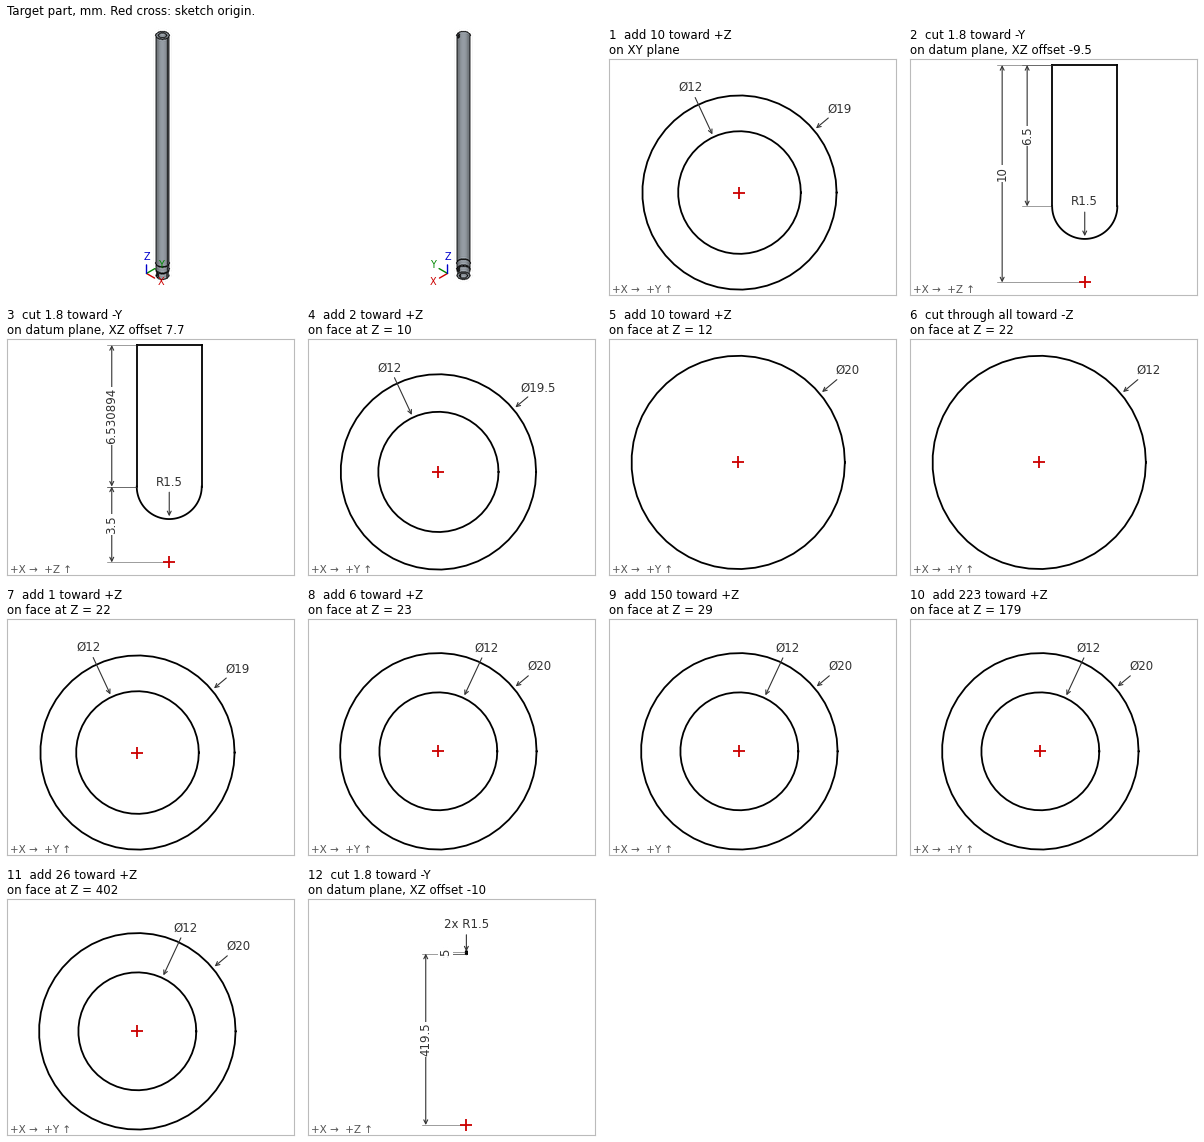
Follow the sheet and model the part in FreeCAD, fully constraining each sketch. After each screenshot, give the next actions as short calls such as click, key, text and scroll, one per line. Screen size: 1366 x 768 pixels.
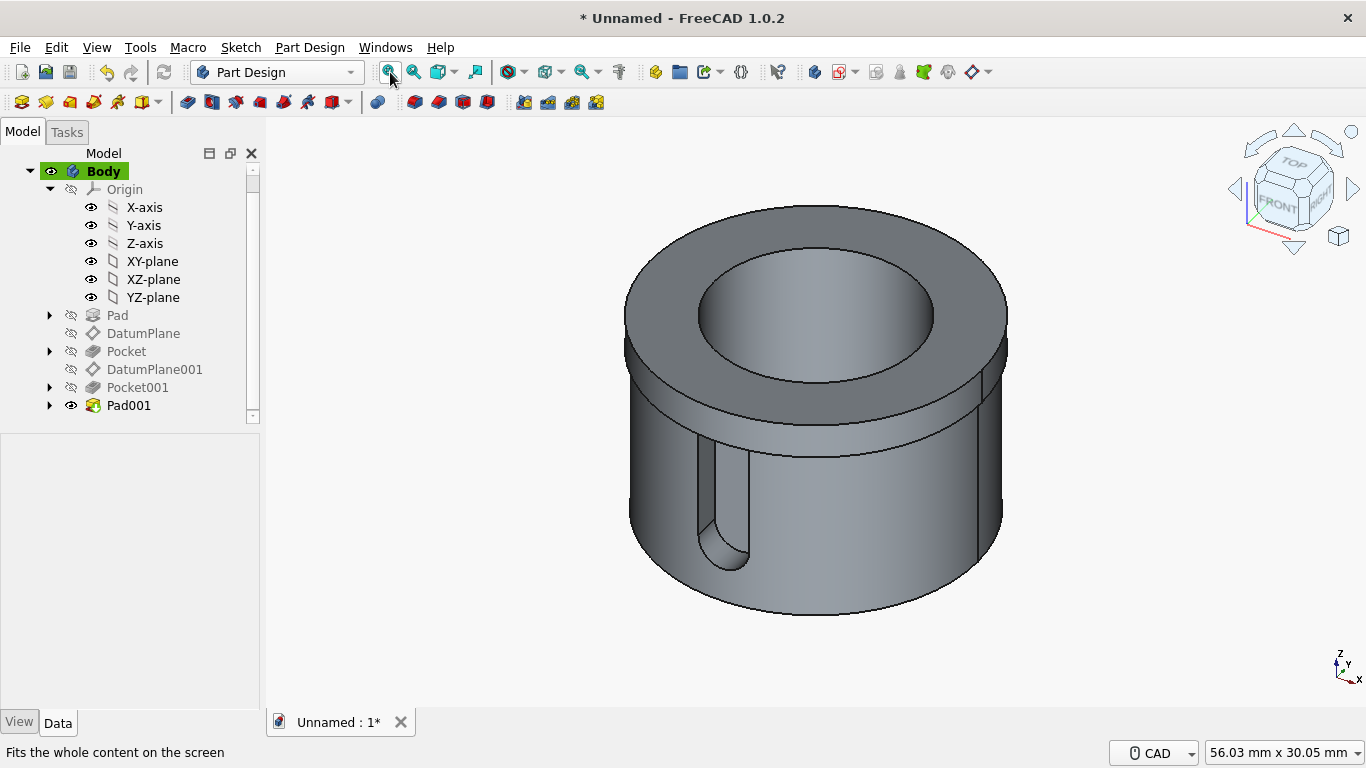
click(965, 292)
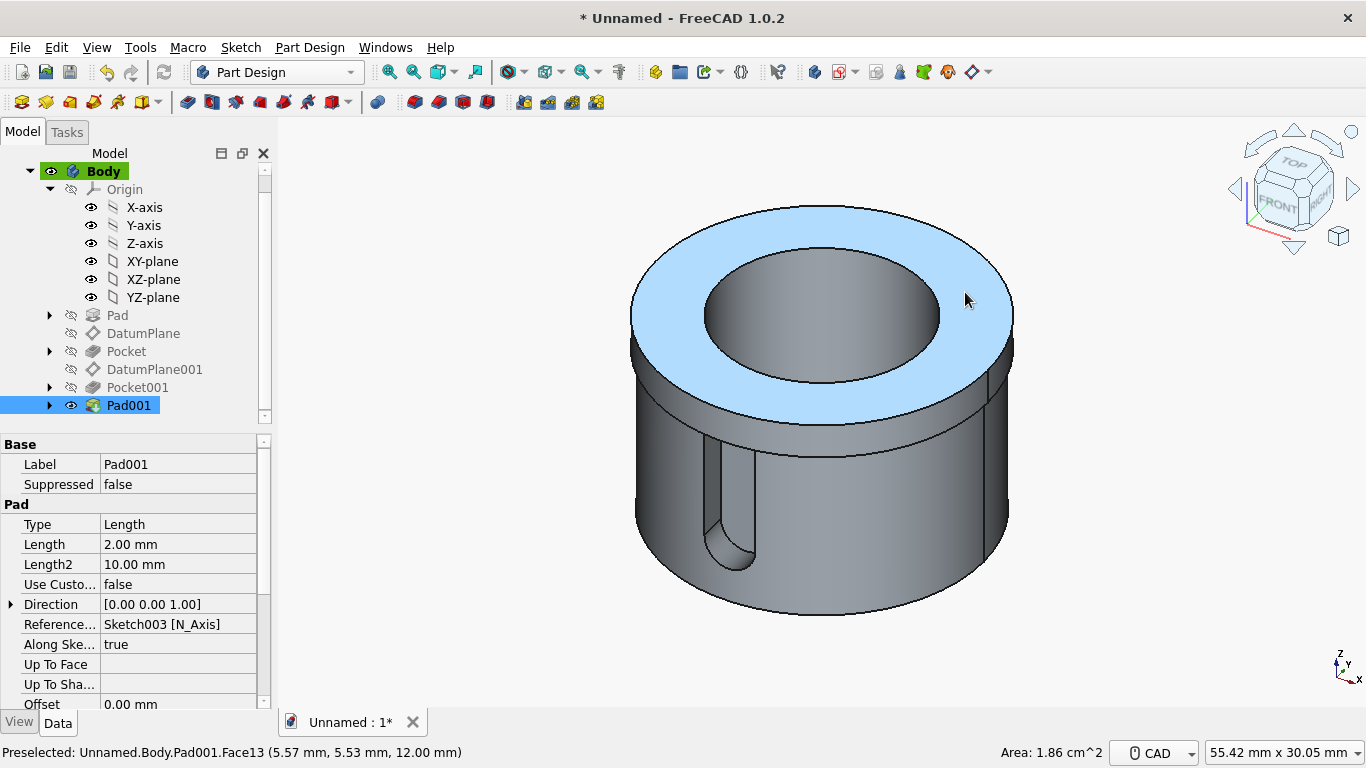
click(840, 72)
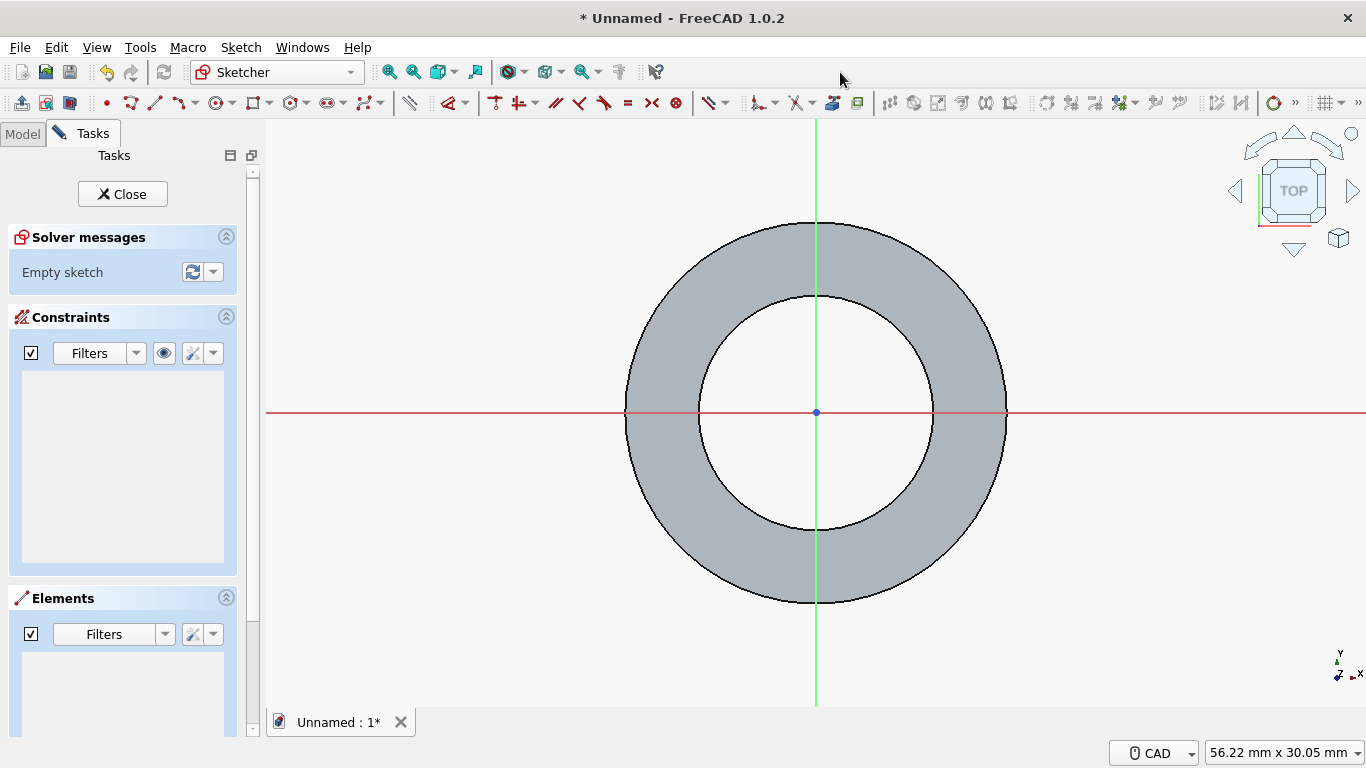
click(216, 104)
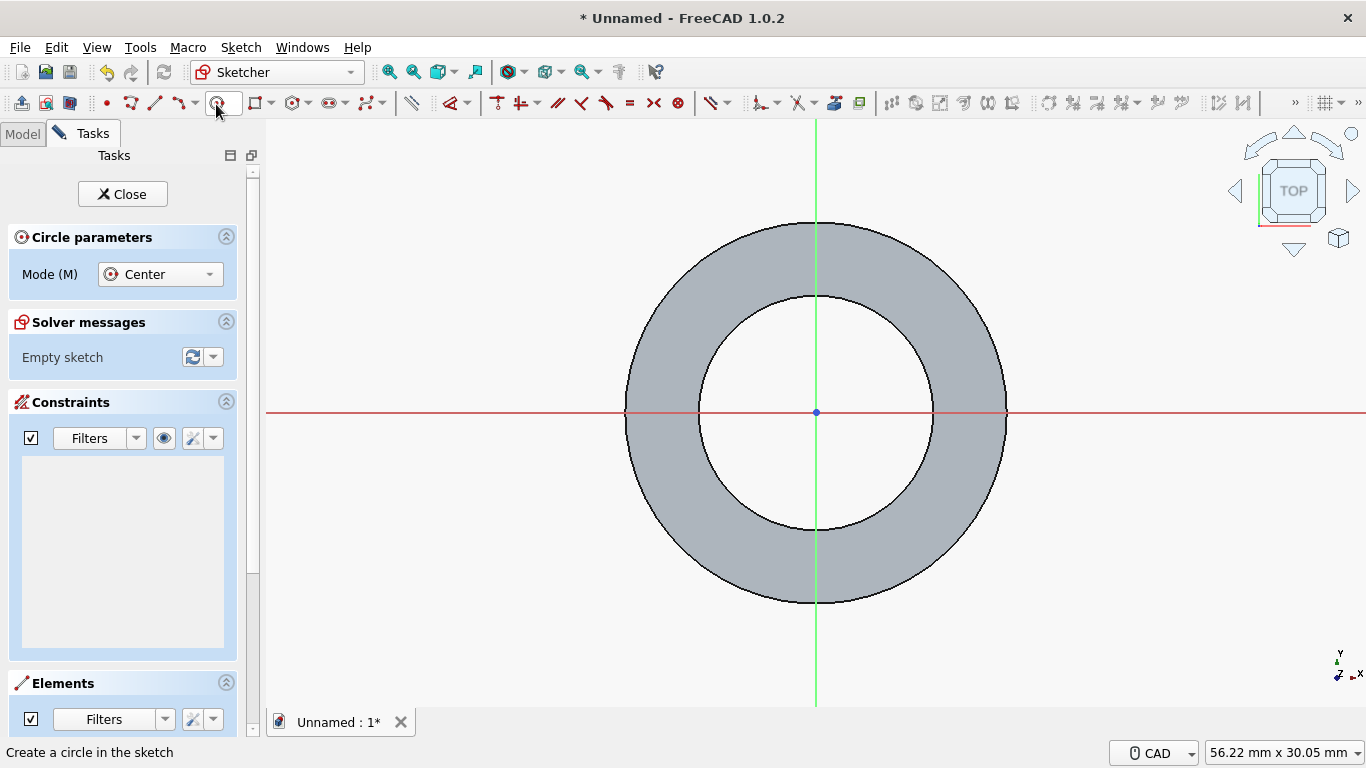
click(816, 413)
click(954, 275)
key(Escape)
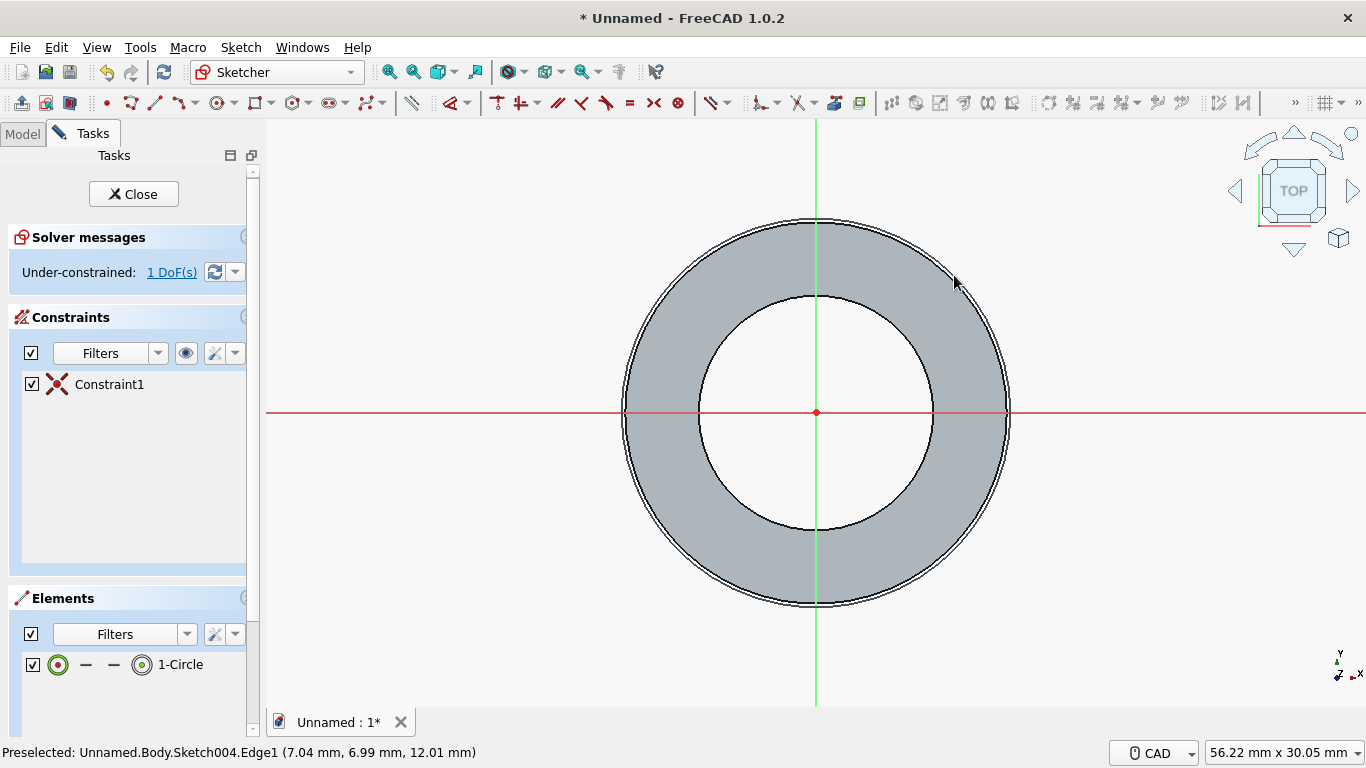
click(450, 104)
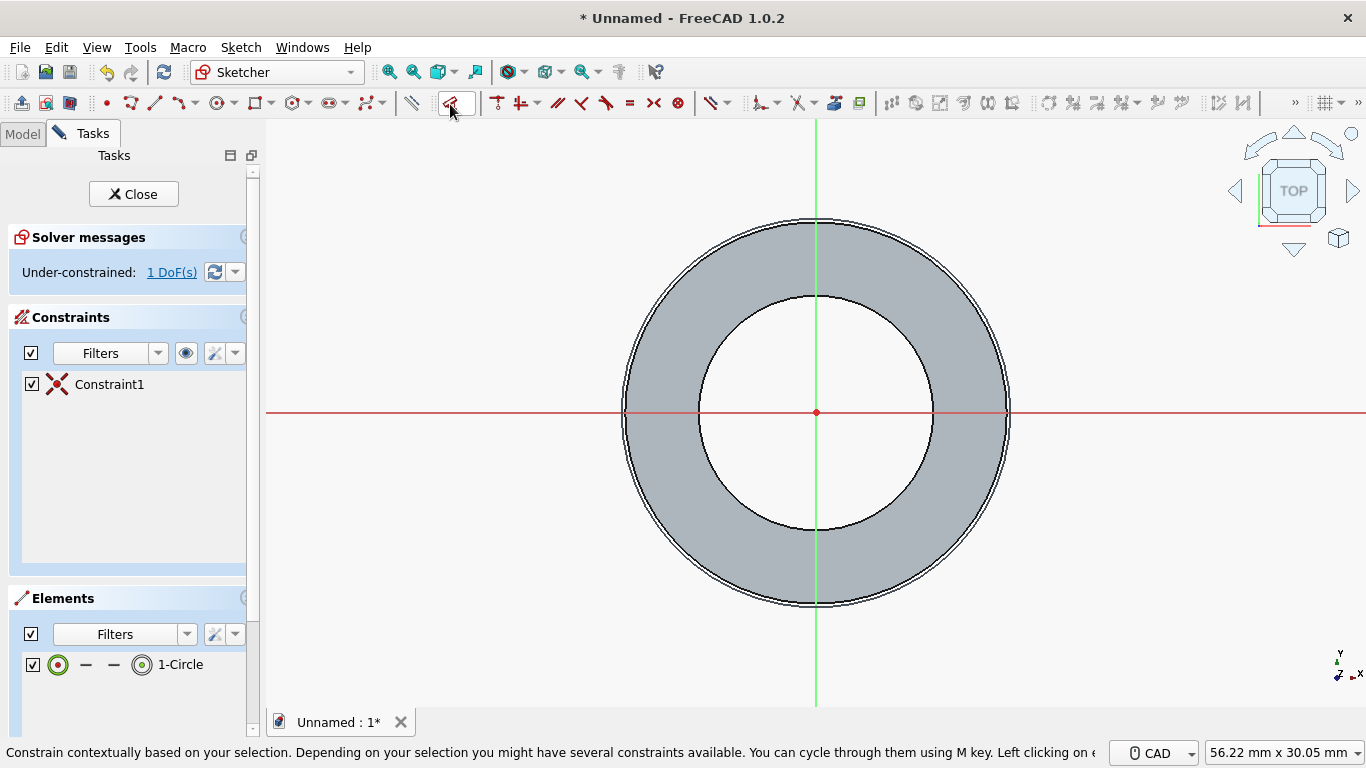
click(953, 275)
click(976, 252)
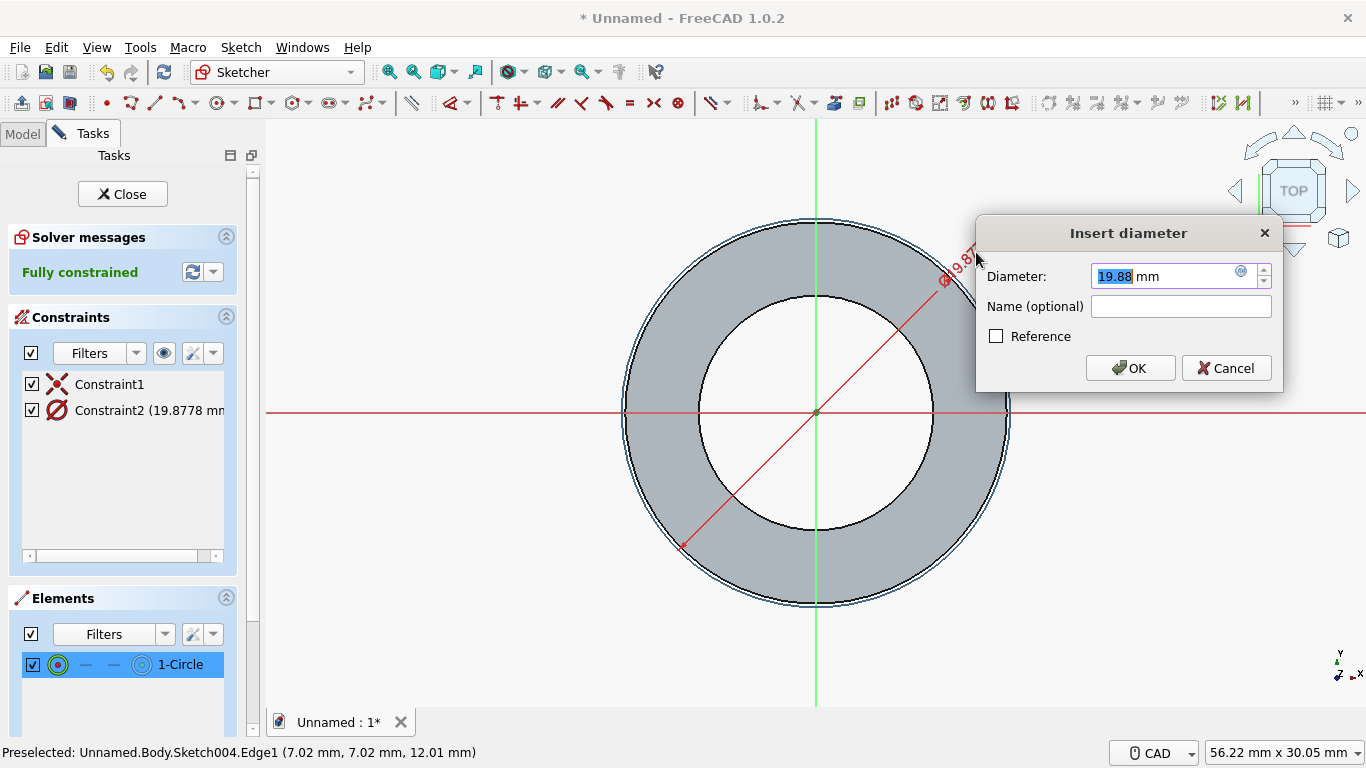
text(20)
key(Return)
key(Escape)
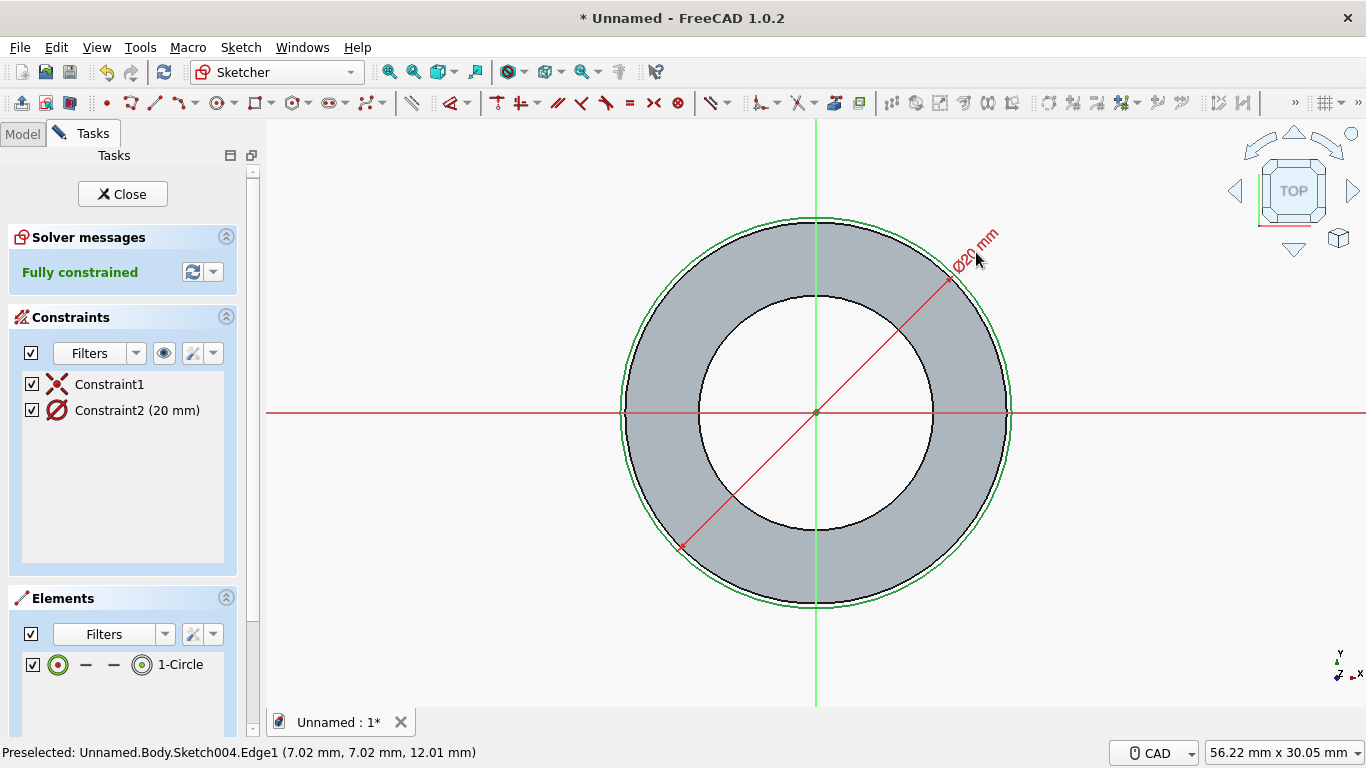
click(123, 194)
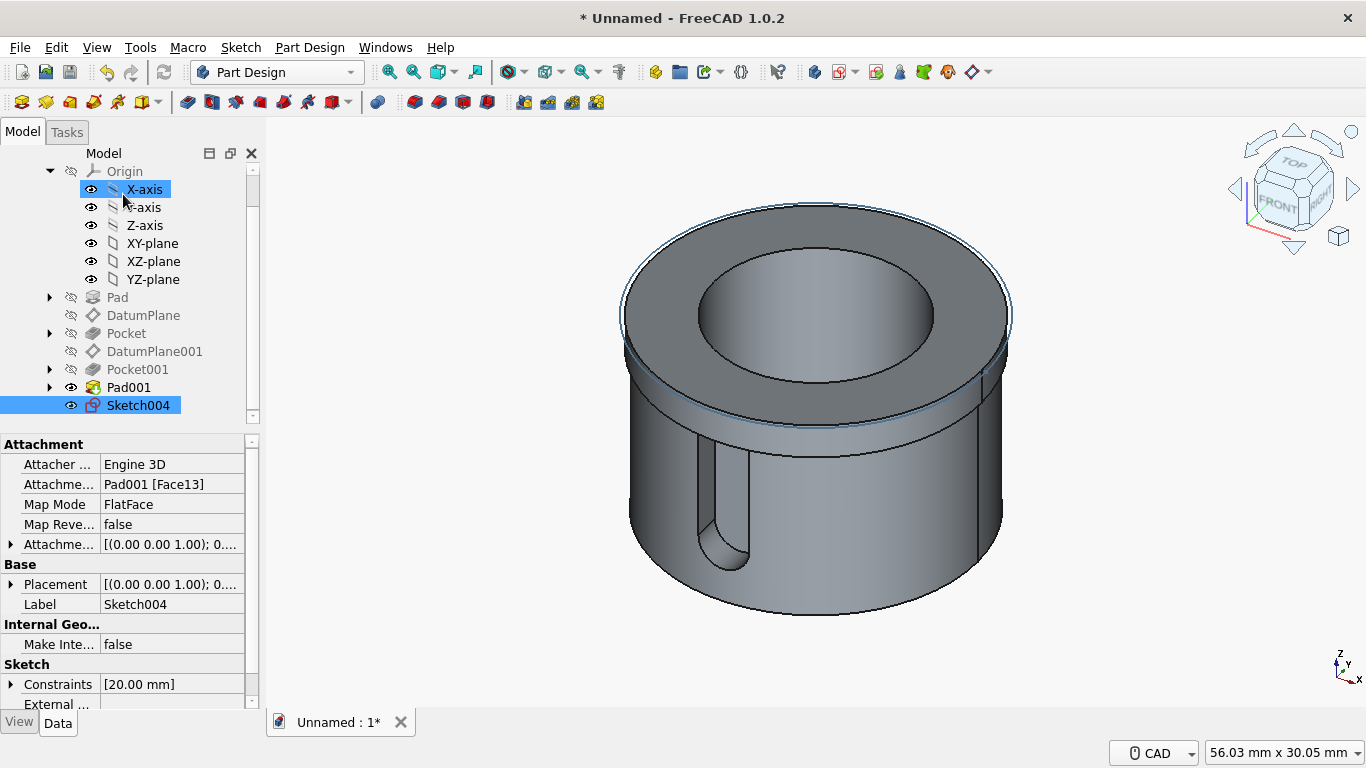
click(22, 102)